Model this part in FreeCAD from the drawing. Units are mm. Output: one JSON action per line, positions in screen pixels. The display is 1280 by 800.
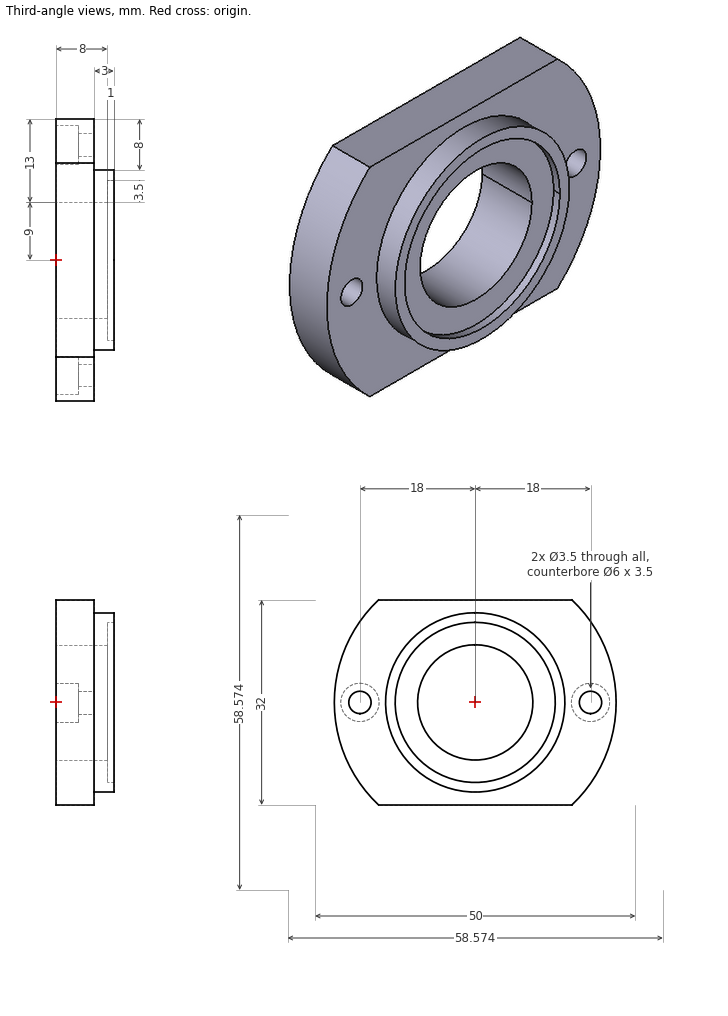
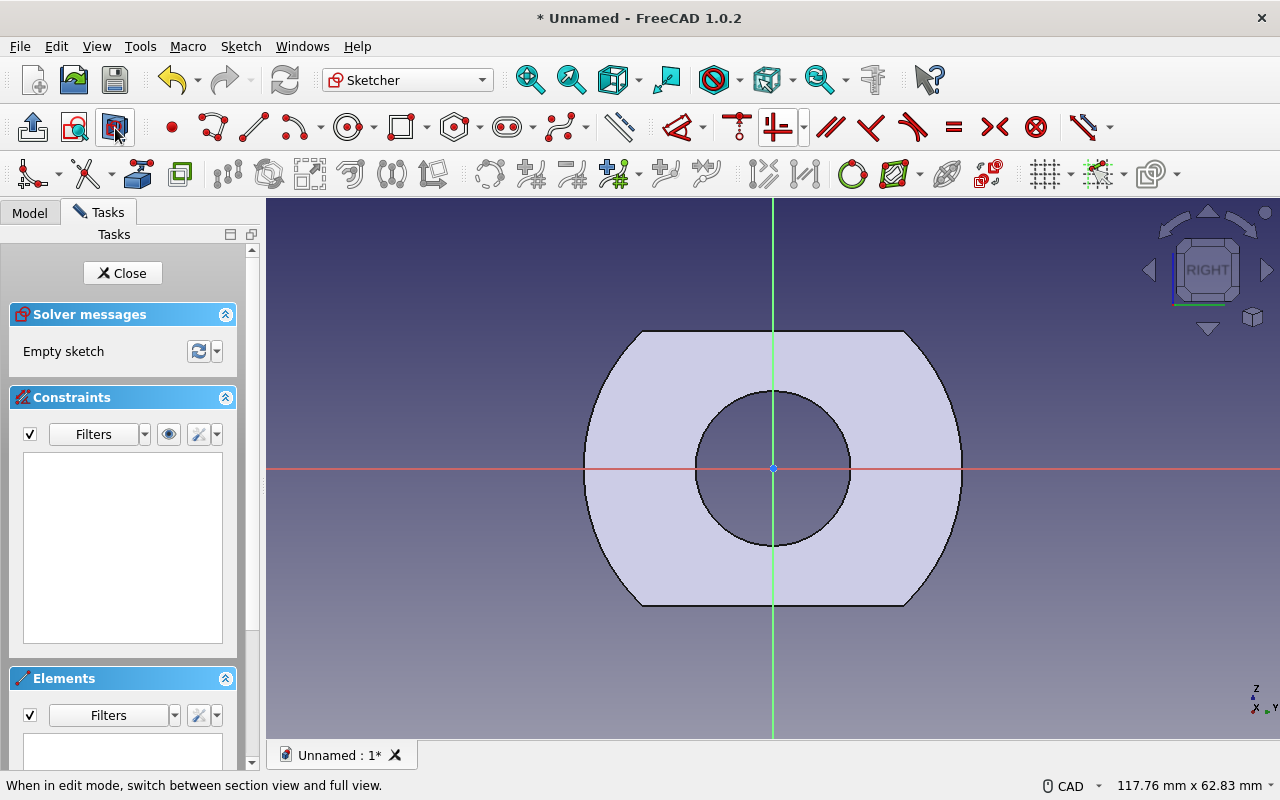
{"action": "scroll", "coordinate": [856, 469], "scroll_direction": "up", "scroll_amount": 3}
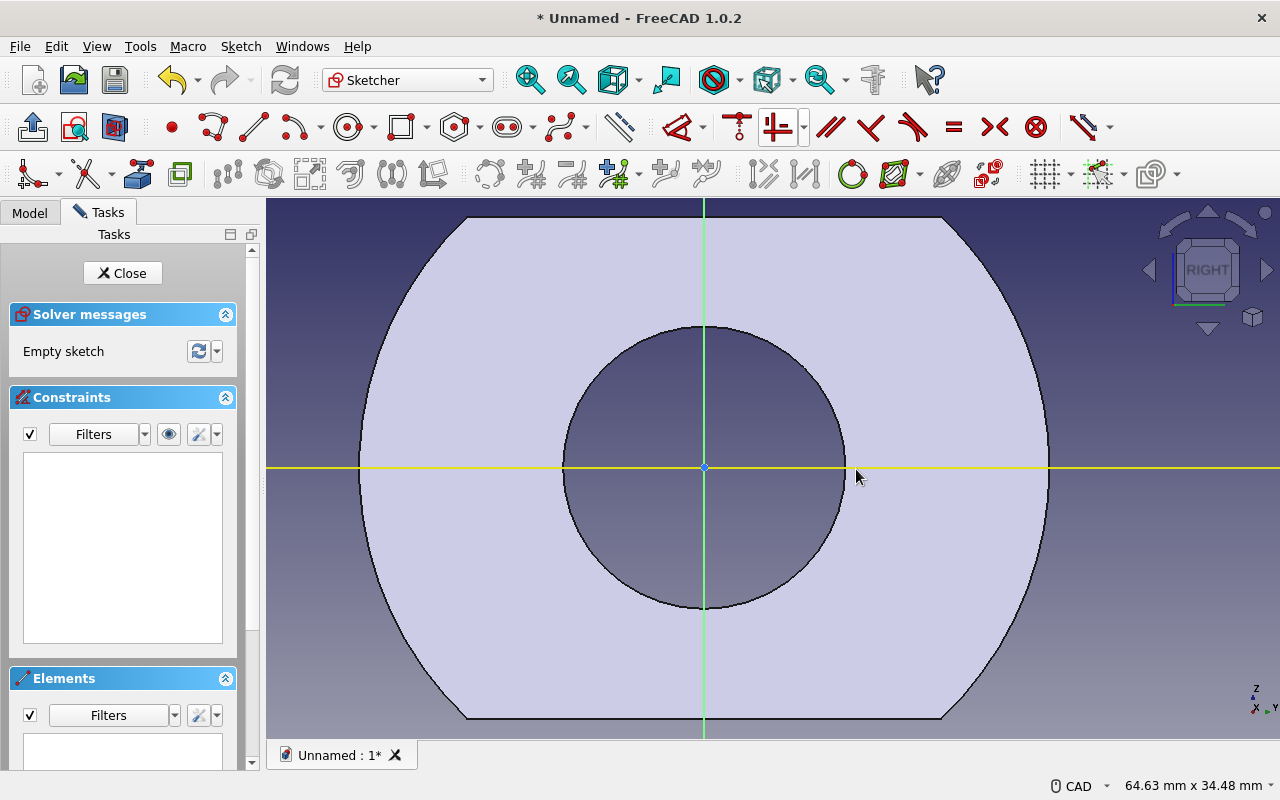
{"action": "left_click", "coordinate": [348, 128]}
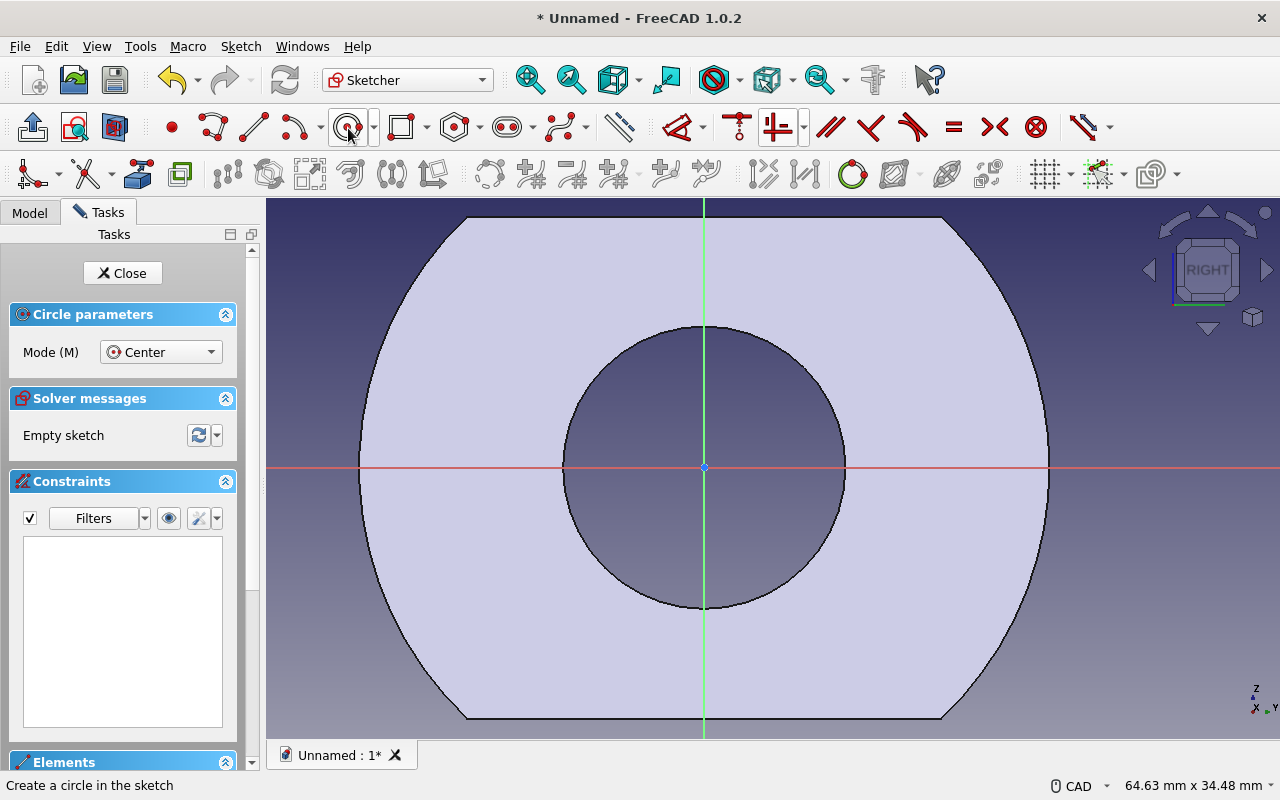
{"action": "left_click", "coordinate": [987, 468]}
{"action": "mouse_move", "coordinate": [1006, 448]}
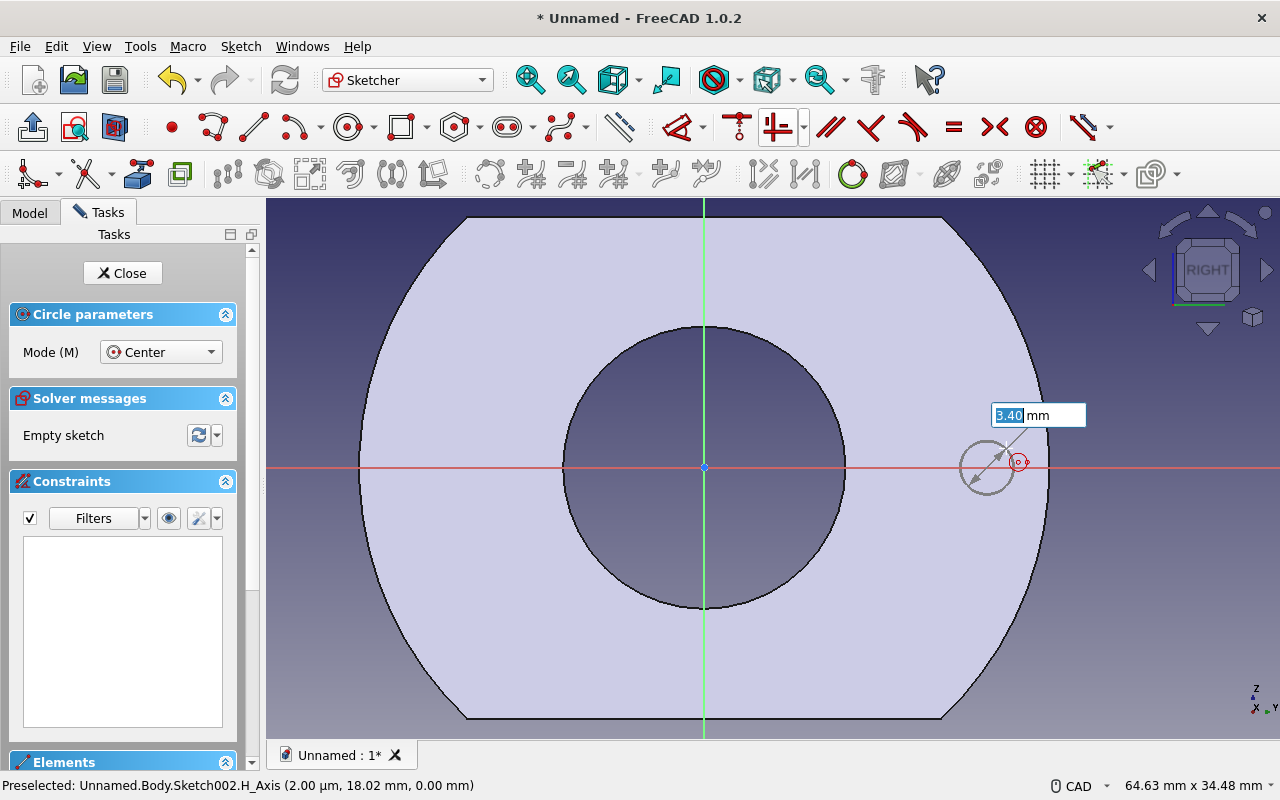
{"action": "type", "text": "3.5"}
{"action": "key", "text": "Return"}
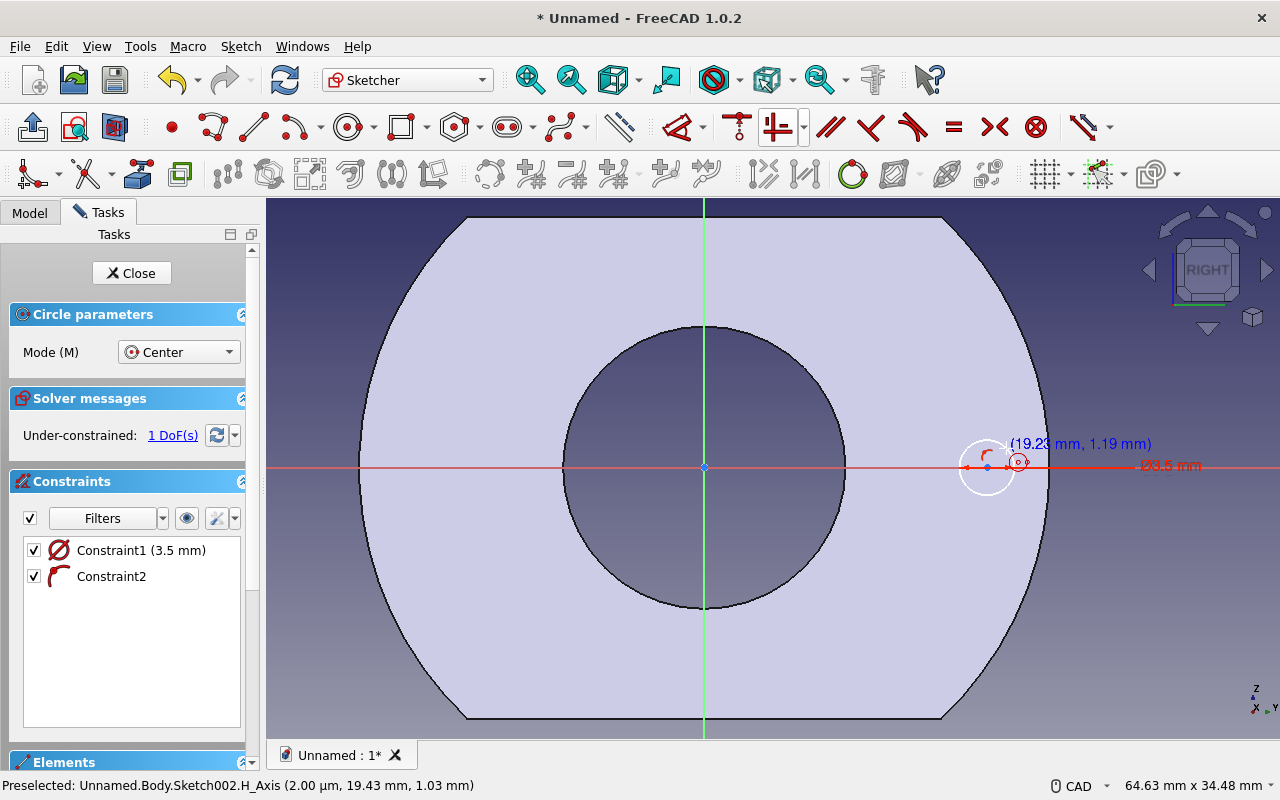
{"action": "left_click", "coordinate": [422, 468]}
{"action": "mouse_move", "coordinate": [441, 448]}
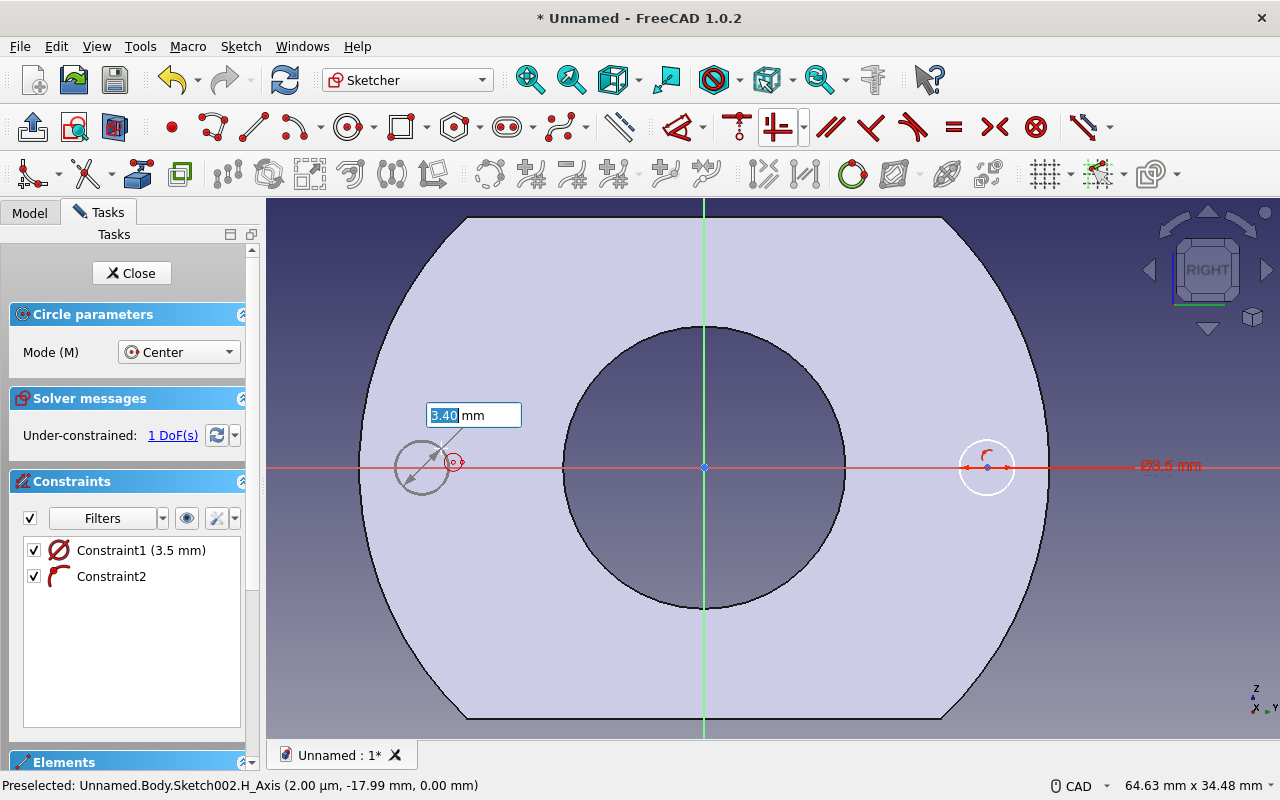
{"action": "type", "text": "3.5"}
{"action": "key", "text": "Return"}
{"action": "key", "text": "Escape"}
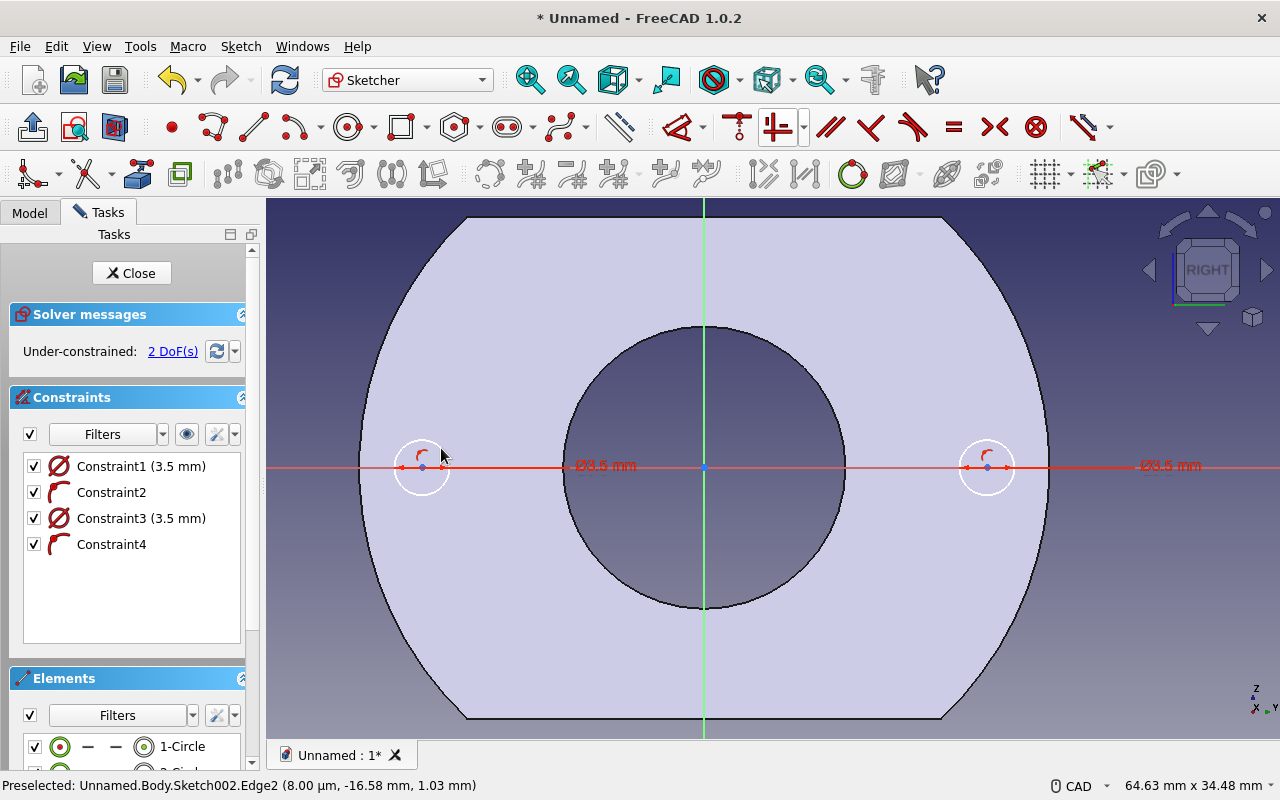
{"action": "left_click", "coordinate": [676, 128]}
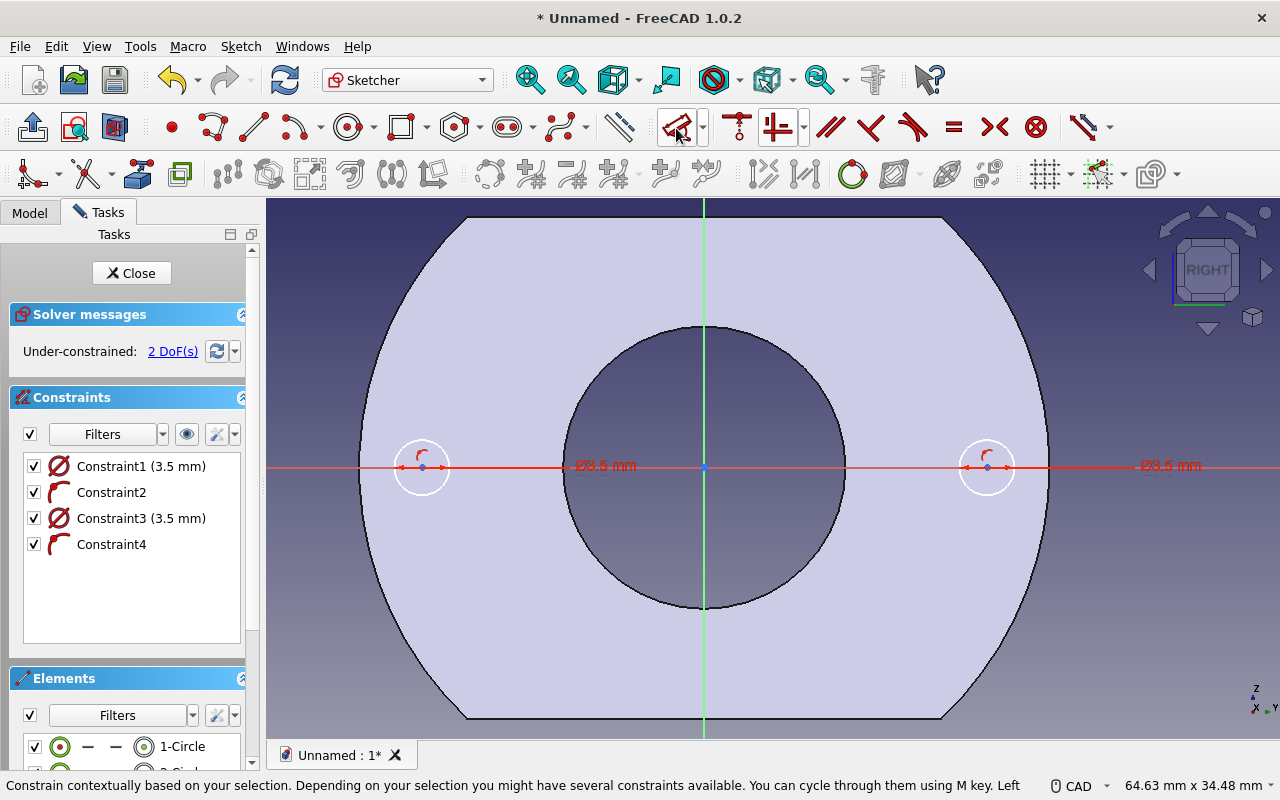
{"action": "left_click", "coordinate": [987, 468]}
{"action": "left_click", "coordinate": [846, 502]}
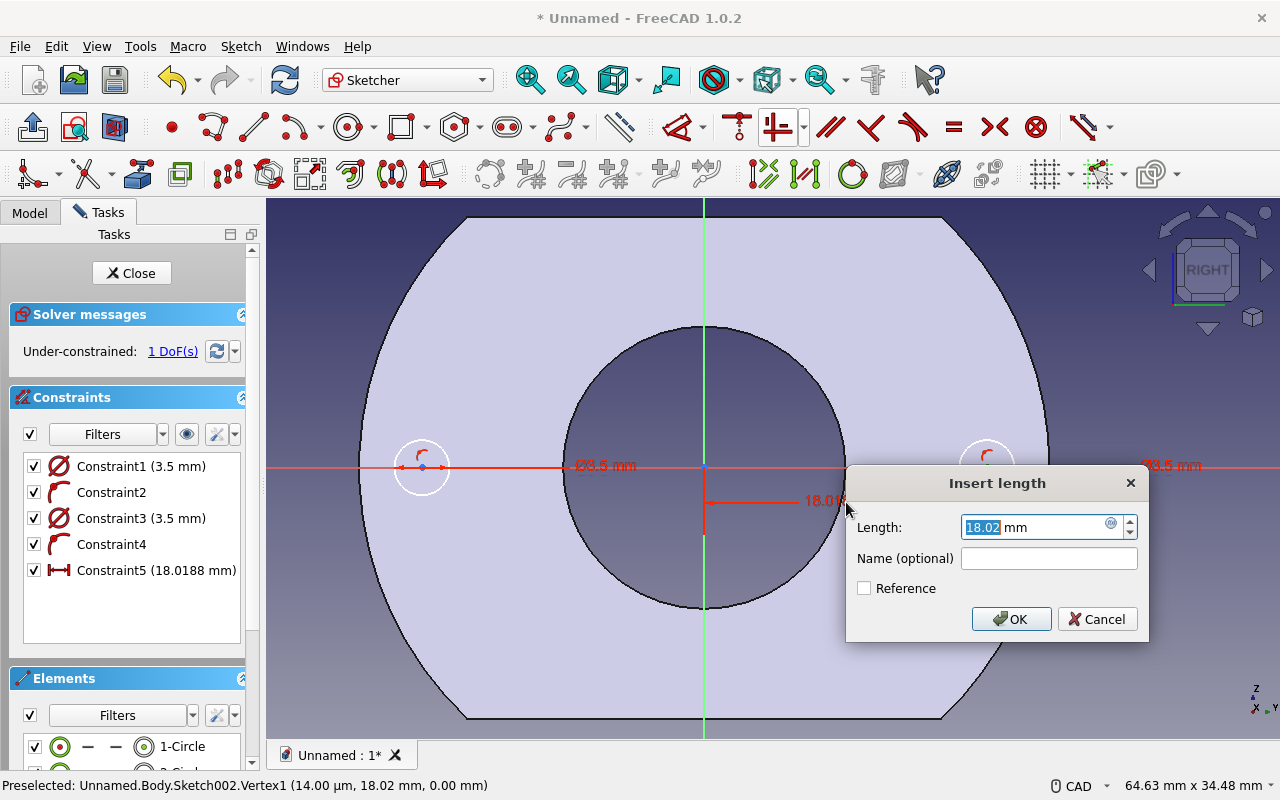
{"action": "type", "text": "18"}
{"action": "key", "text": "Return"}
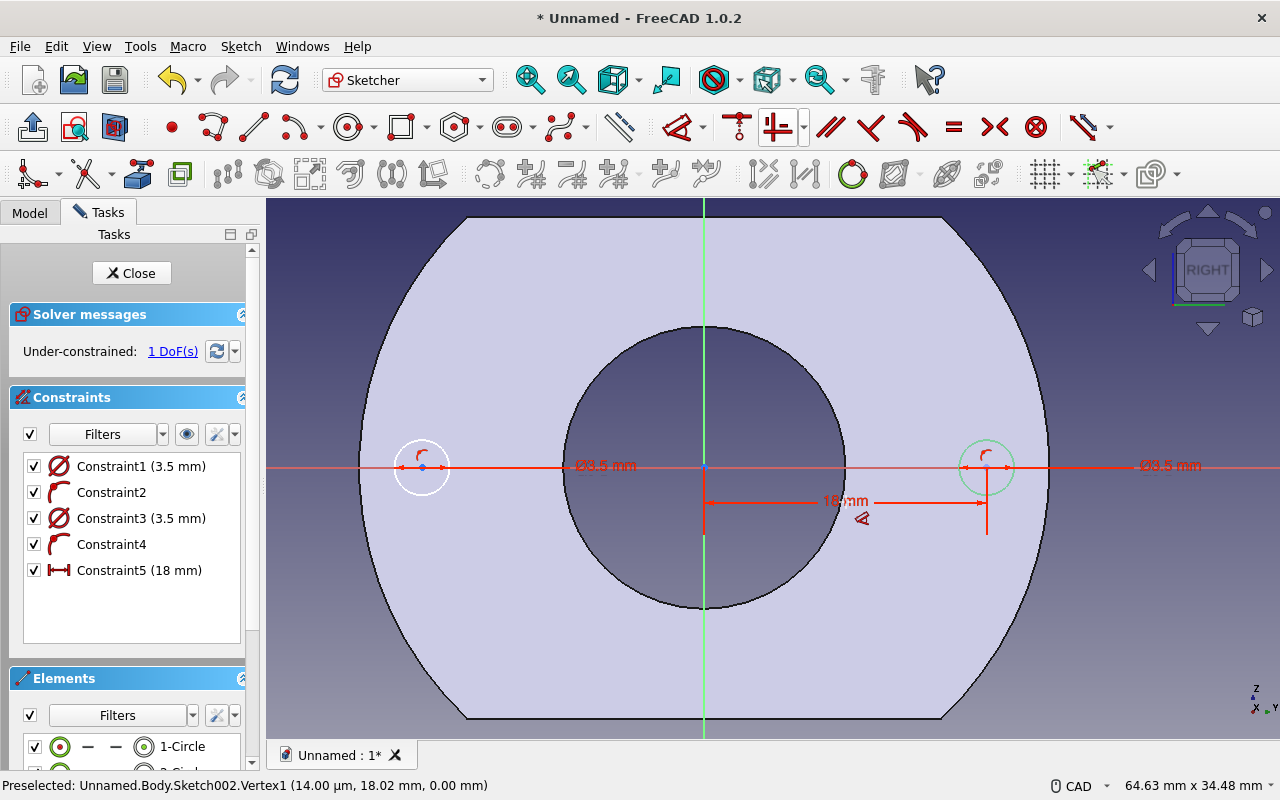
{"action": "left_click", "coordinate": [422, 468]}
{"action": "left_click", "coordinate": [563, 502]}